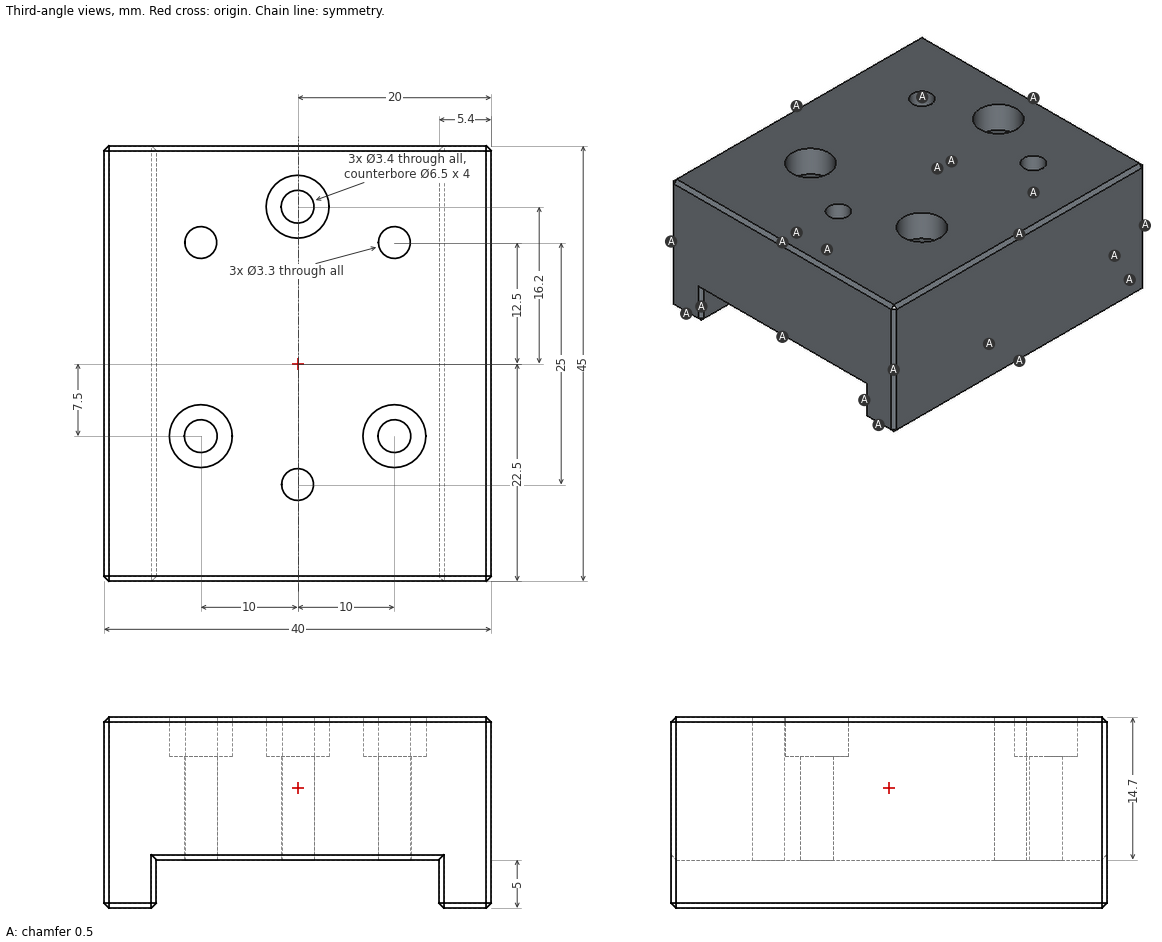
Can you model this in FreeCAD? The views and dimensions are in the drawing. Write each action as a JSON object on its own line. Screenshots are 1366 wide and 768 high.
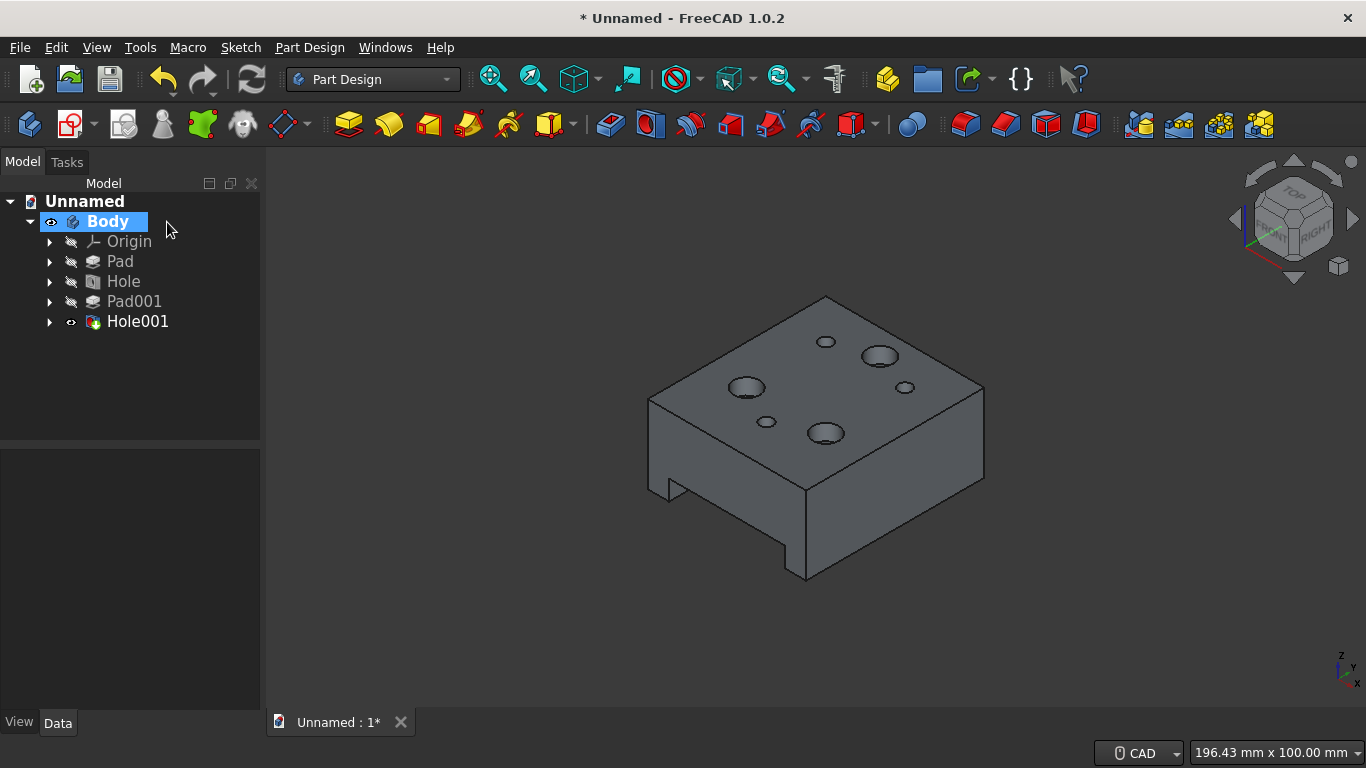
{"action": "left_click", "coordinate": [921, 468]}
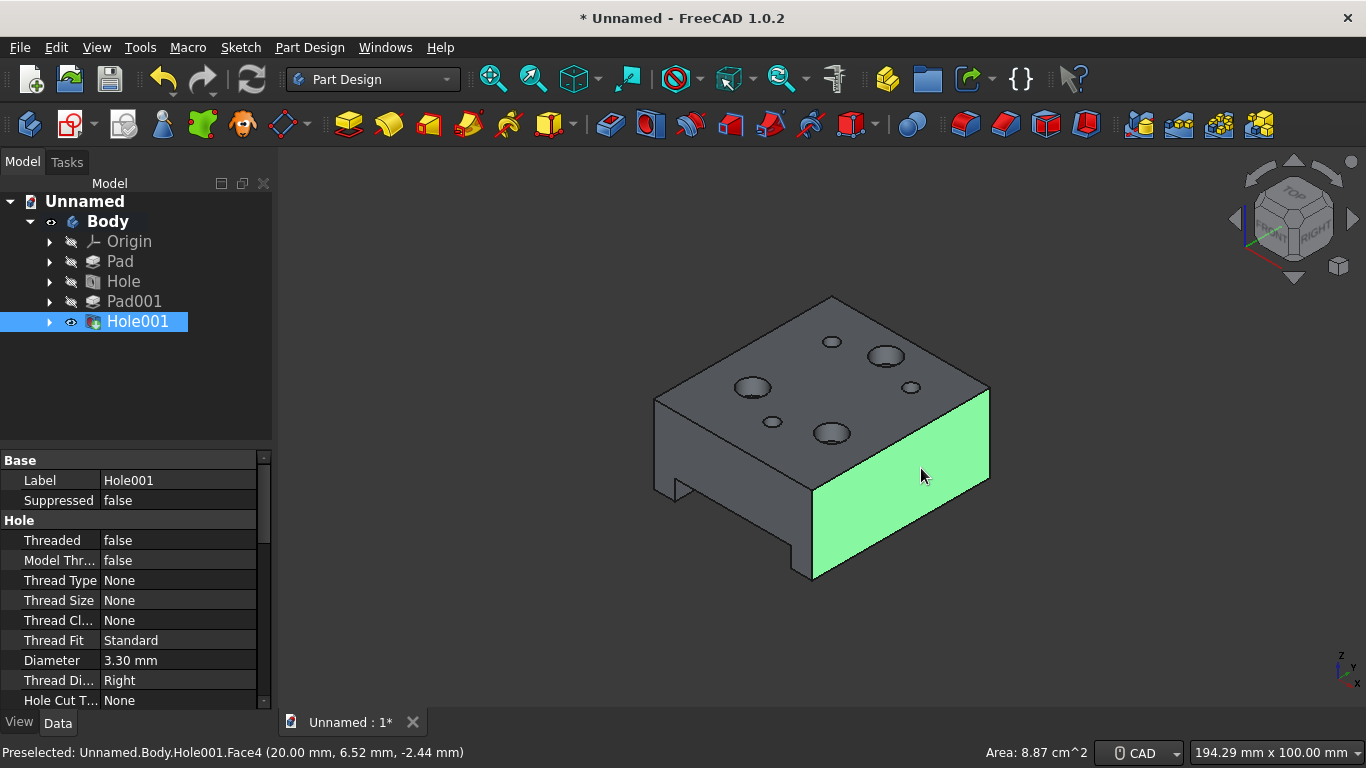
{"action": "left_click", "coordinate": [778, 502], "text": "ctrl"}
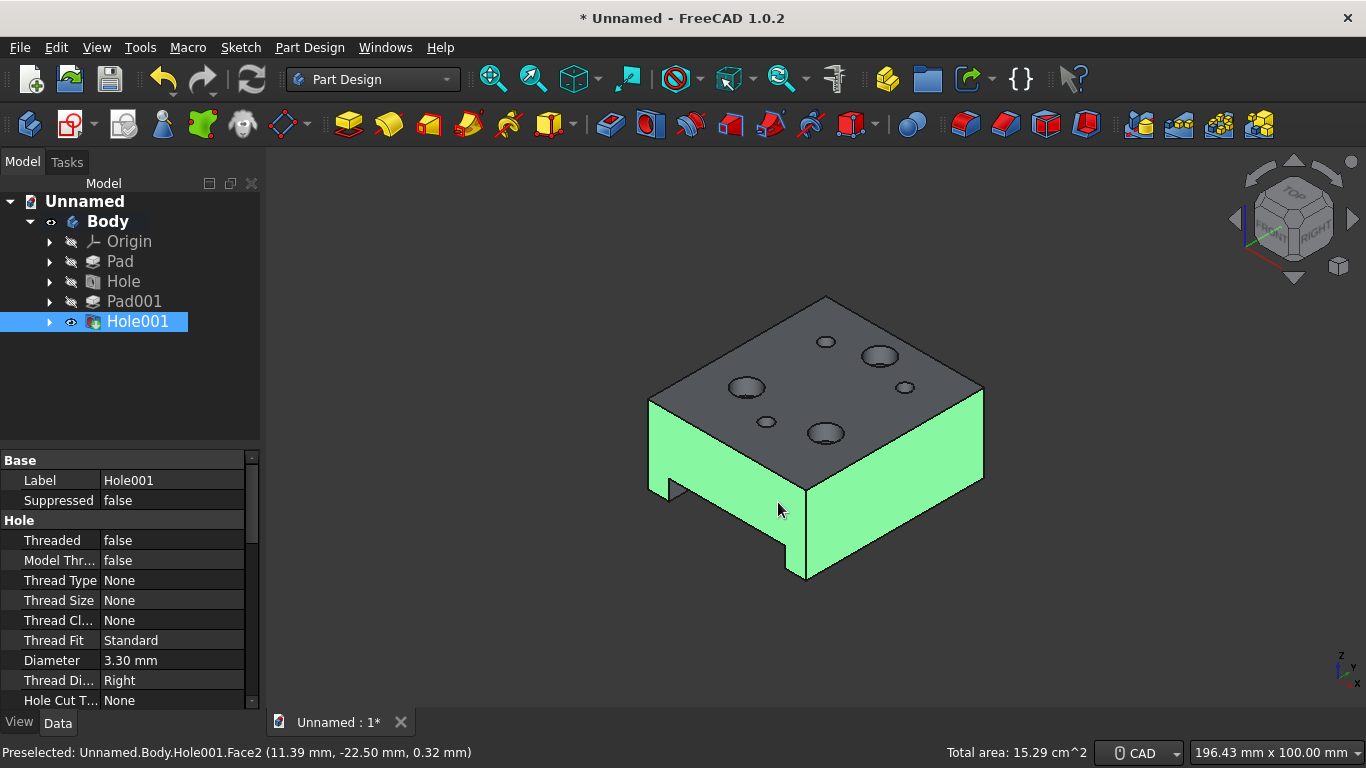
{"action": "key", "text": "2"}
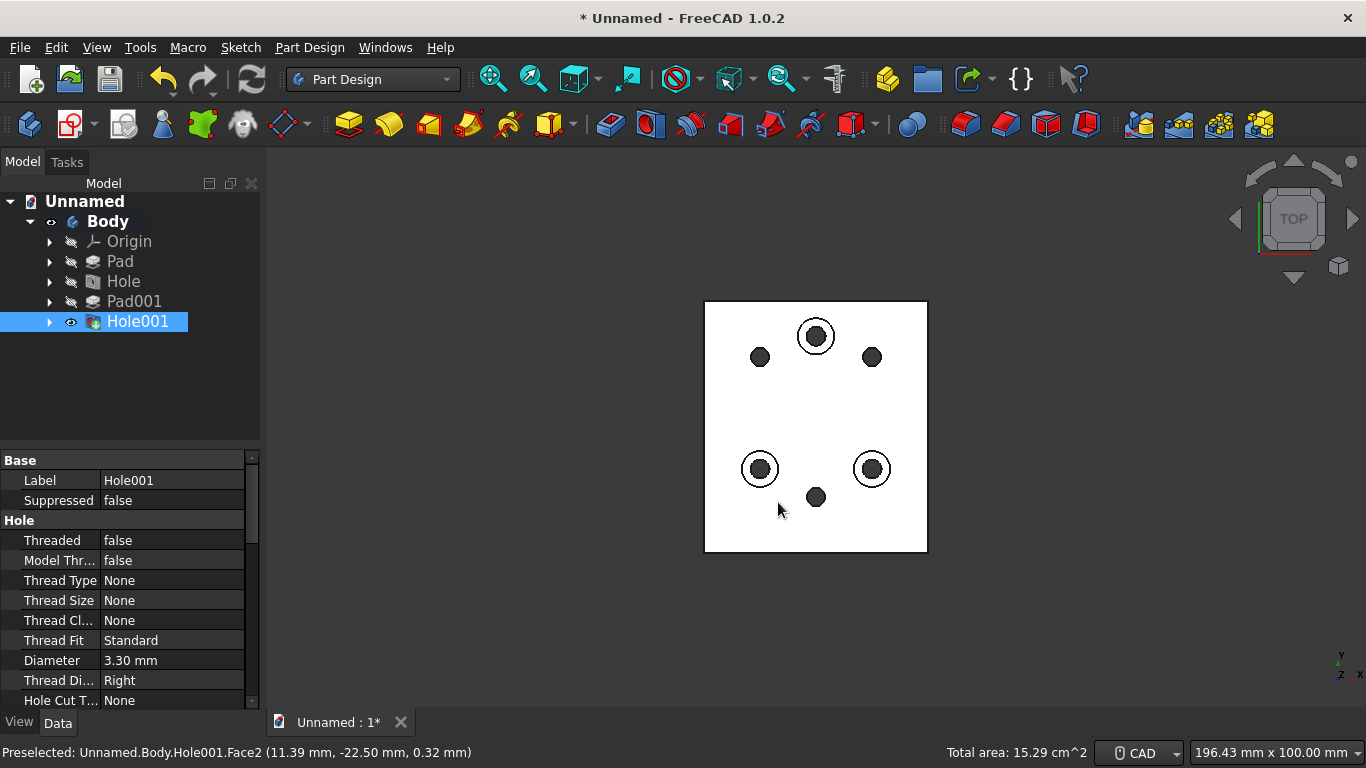
{"action": "key", "text": "0"}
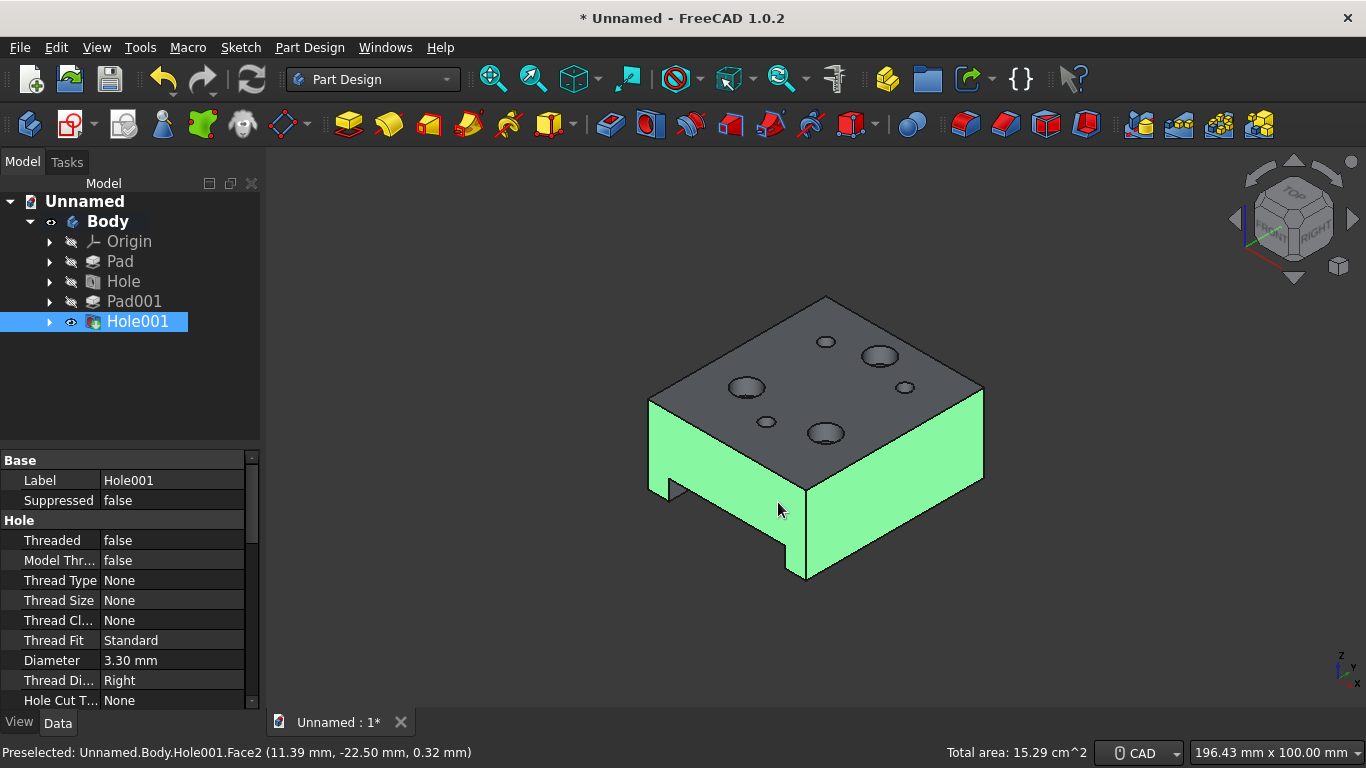
{"action": "key", "text": "1"}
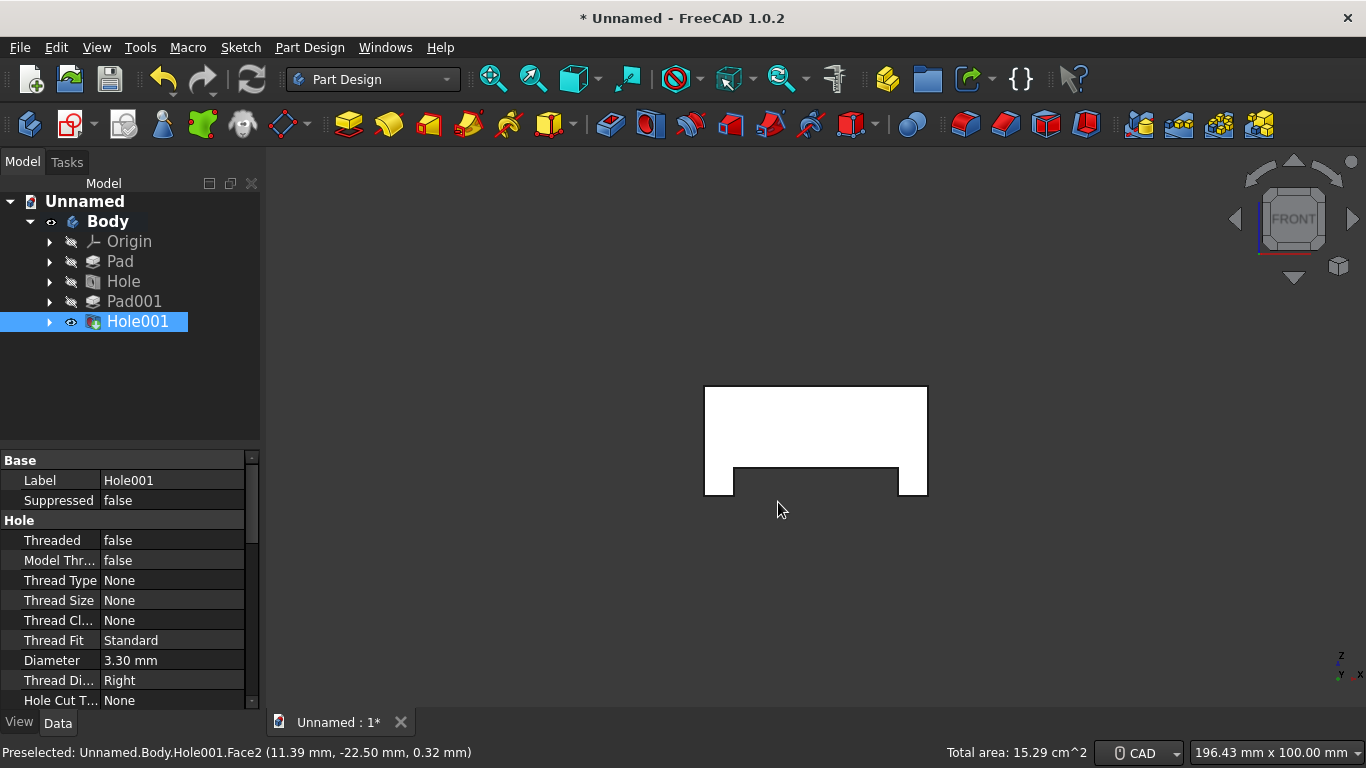
{"action": "left_click", "coordinate": [494, 80]}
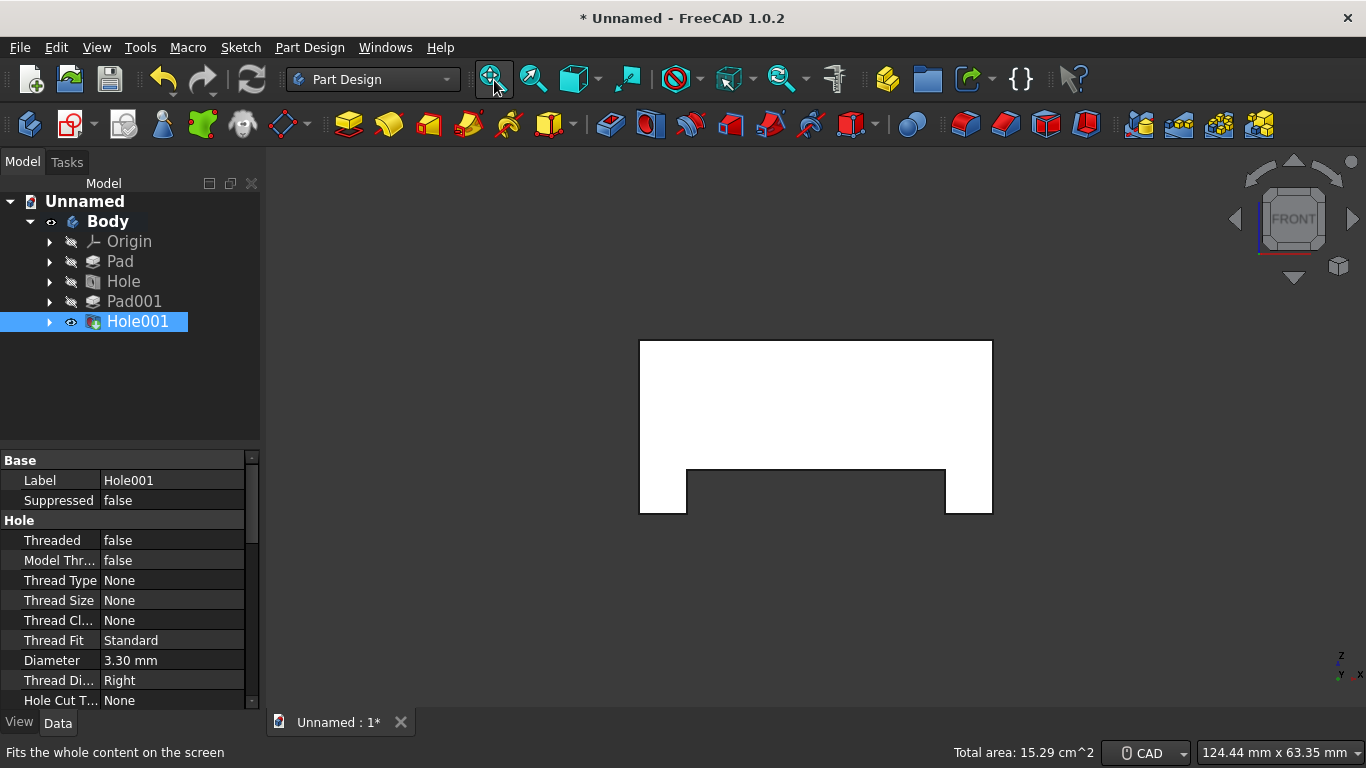
{"action": "key", "text": "3"}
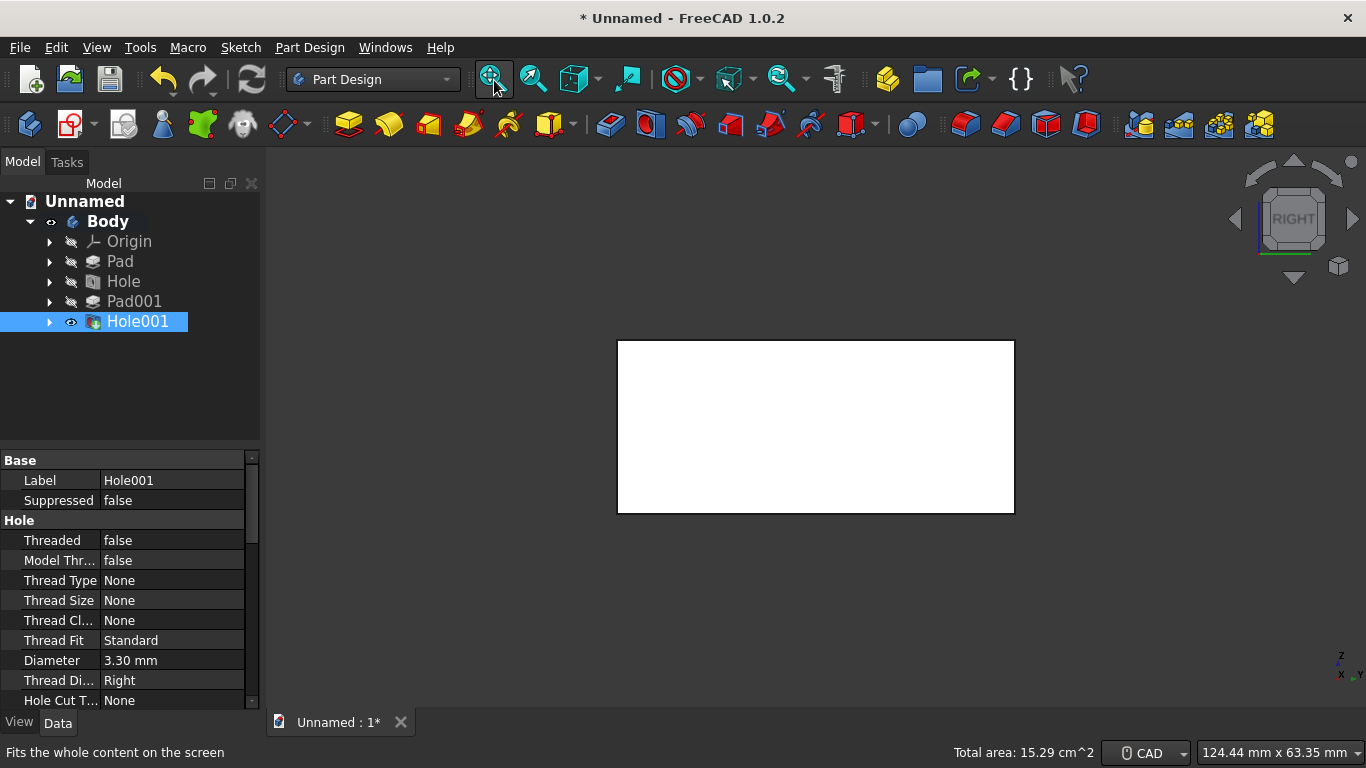
{"action": "left_click", "coordinate": [494, 80]}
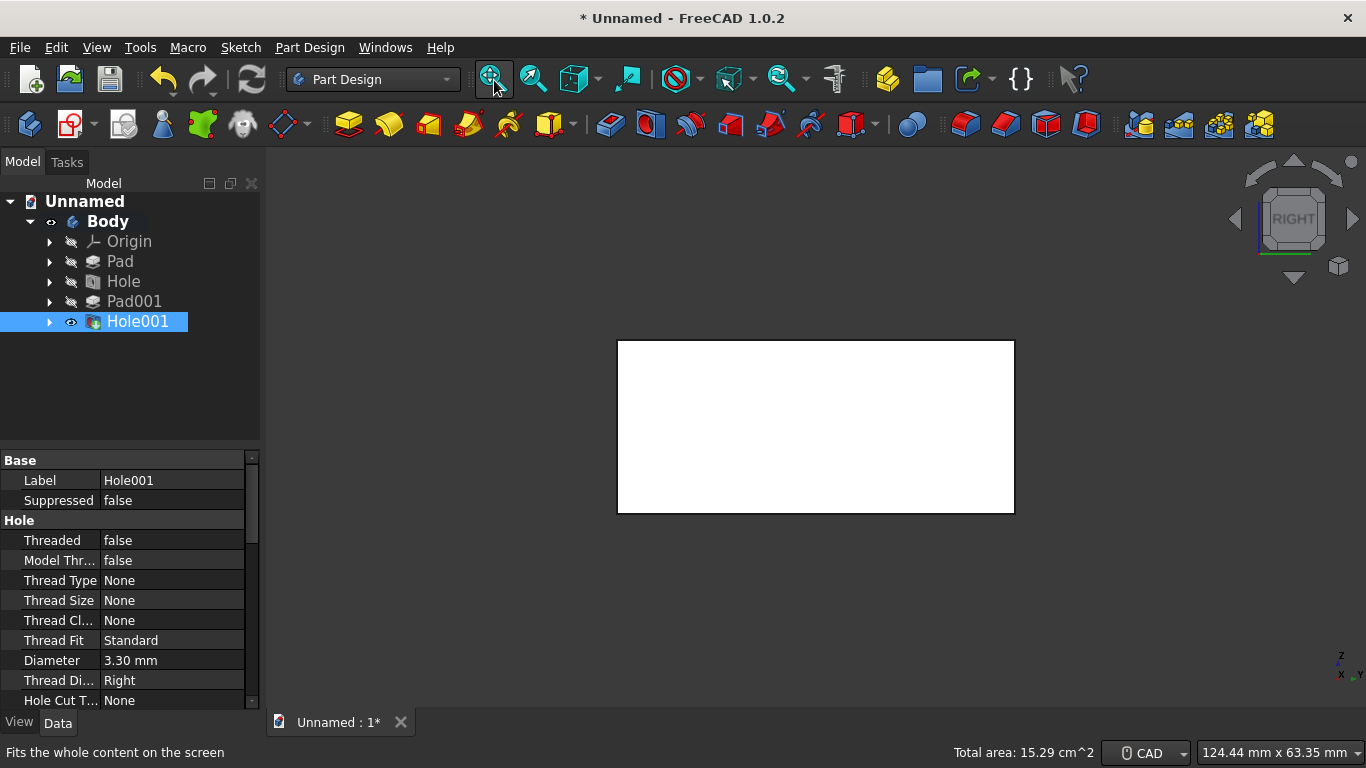
{"action": "key", "text": "5"}